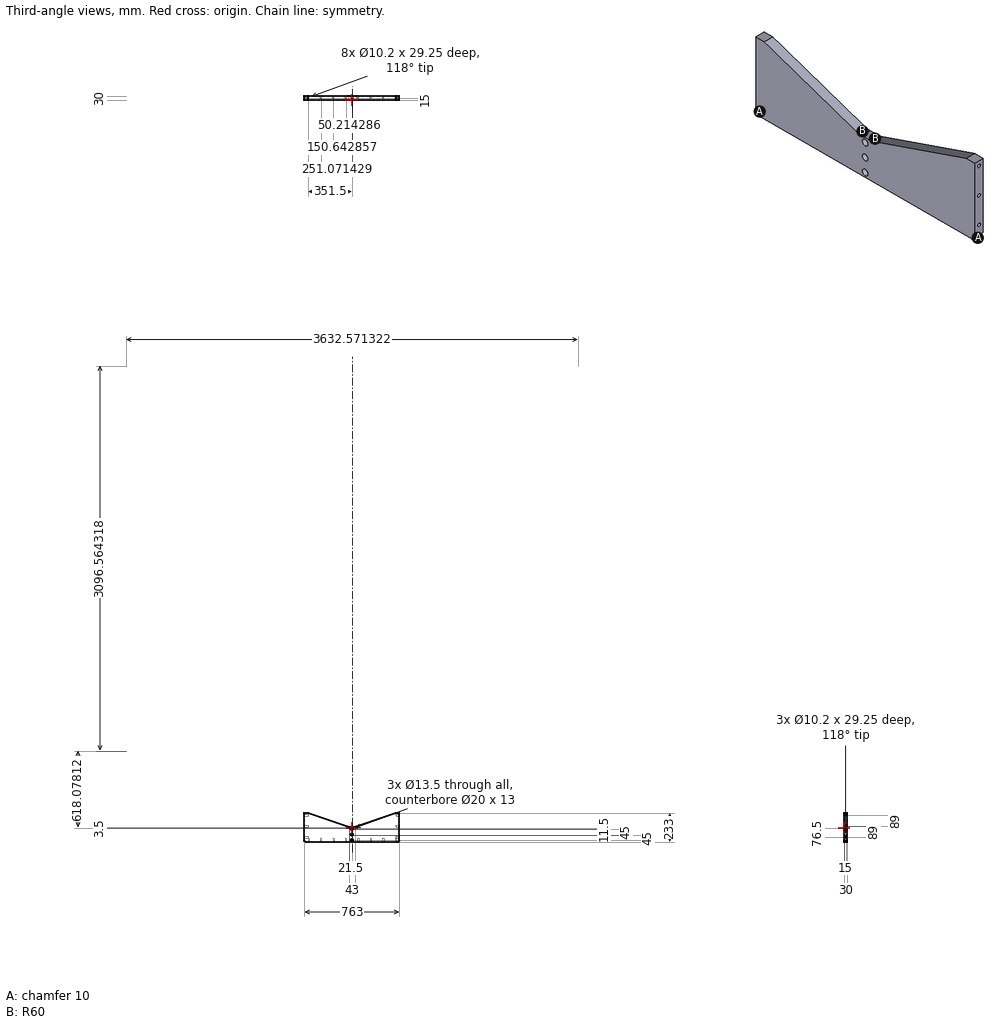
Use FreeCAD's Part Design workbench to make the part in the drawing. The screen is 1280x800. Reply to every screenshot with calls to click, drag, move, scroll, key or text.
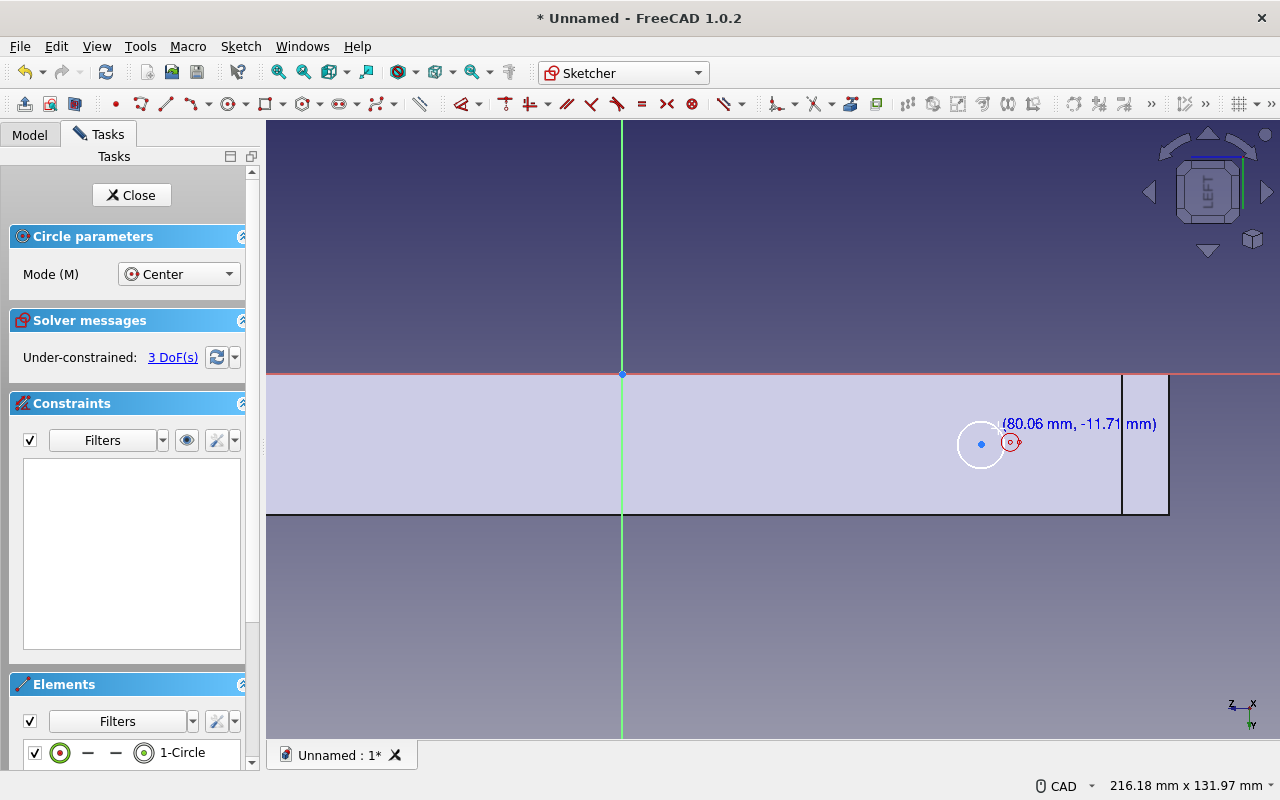
click(564, 444)
click(581, 428)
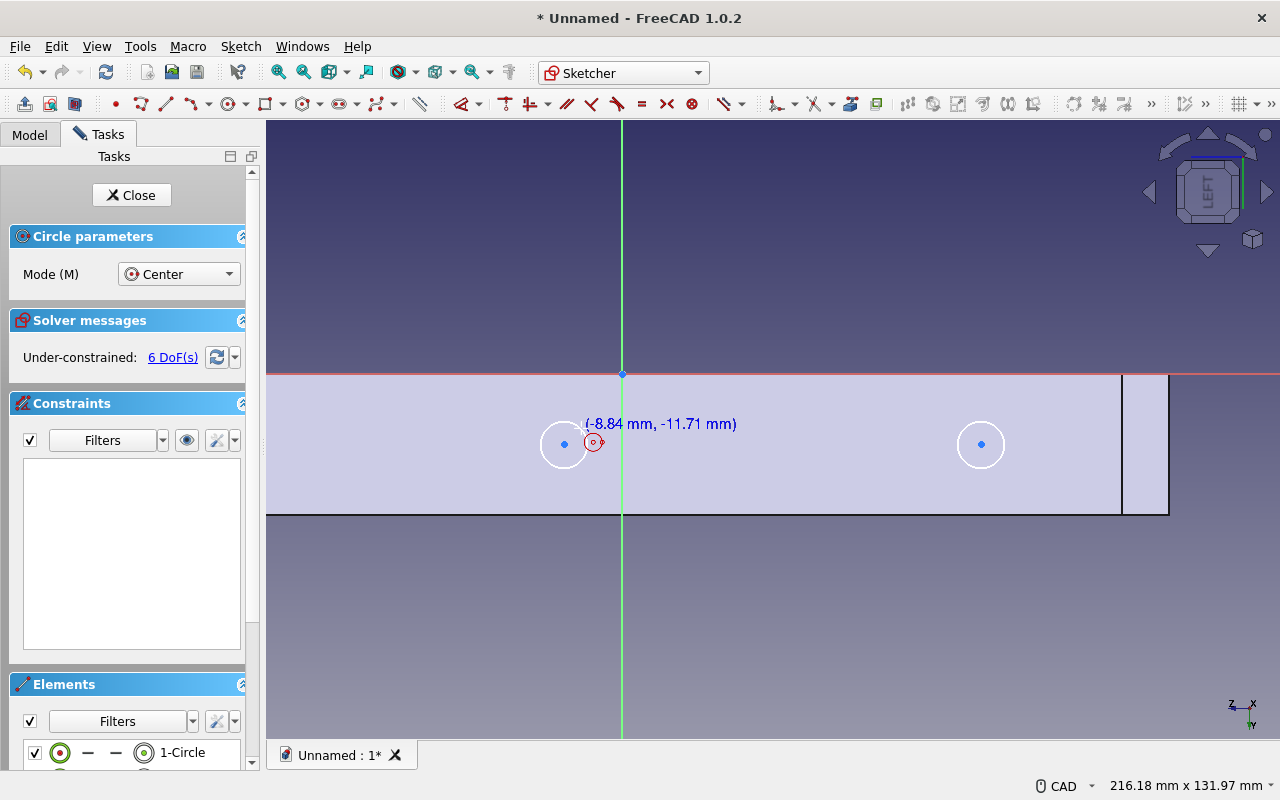
scroll(991, 446, down, 2)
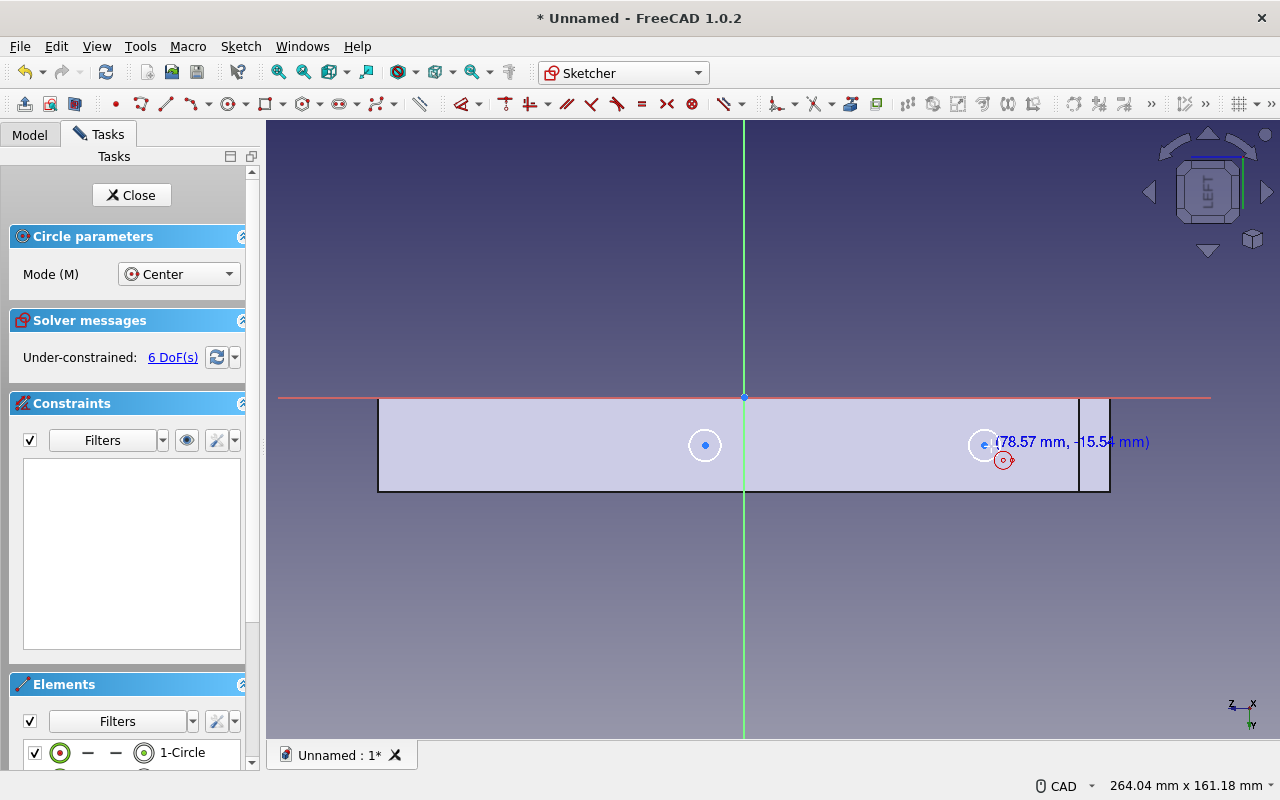
scroll(425, 445, up, 2)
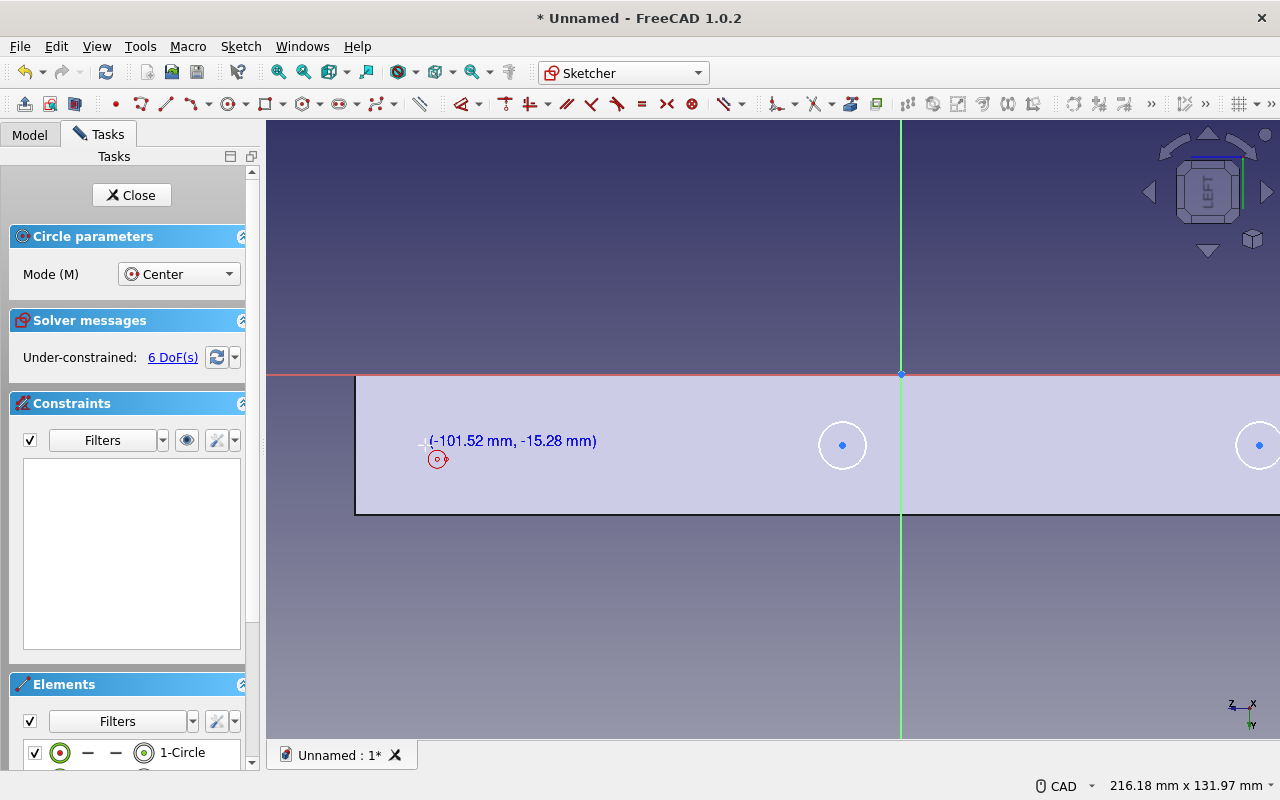
click(425, 445)
click(442, 428)
key(Escape)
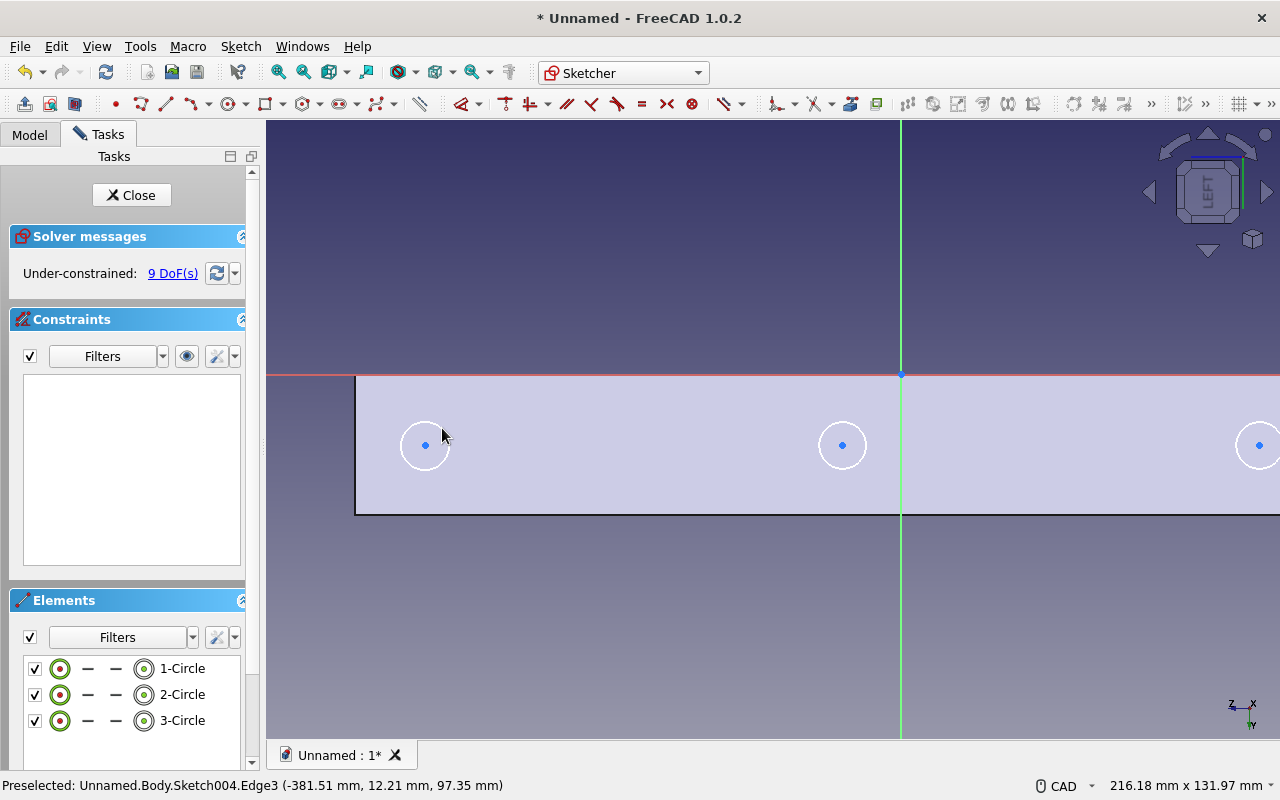
scroll(424, 445, down, 2)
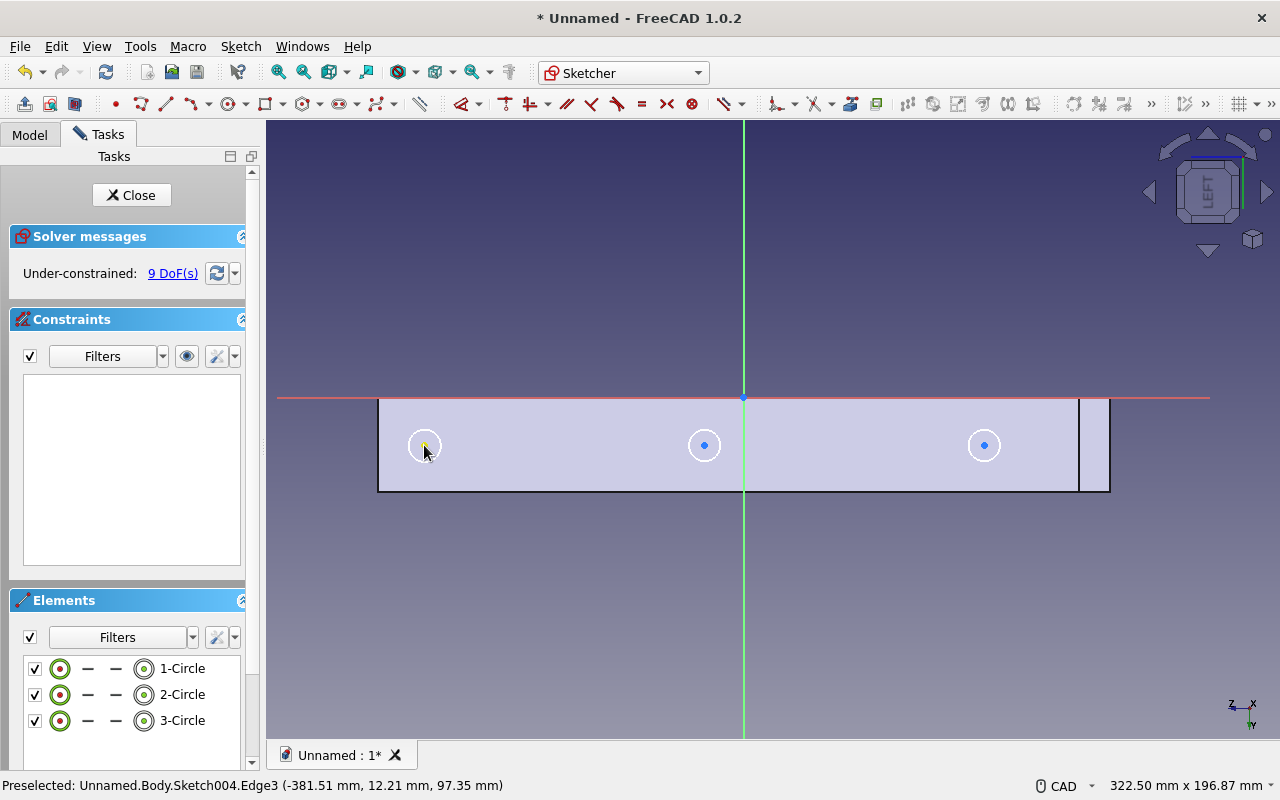
click(995, 434)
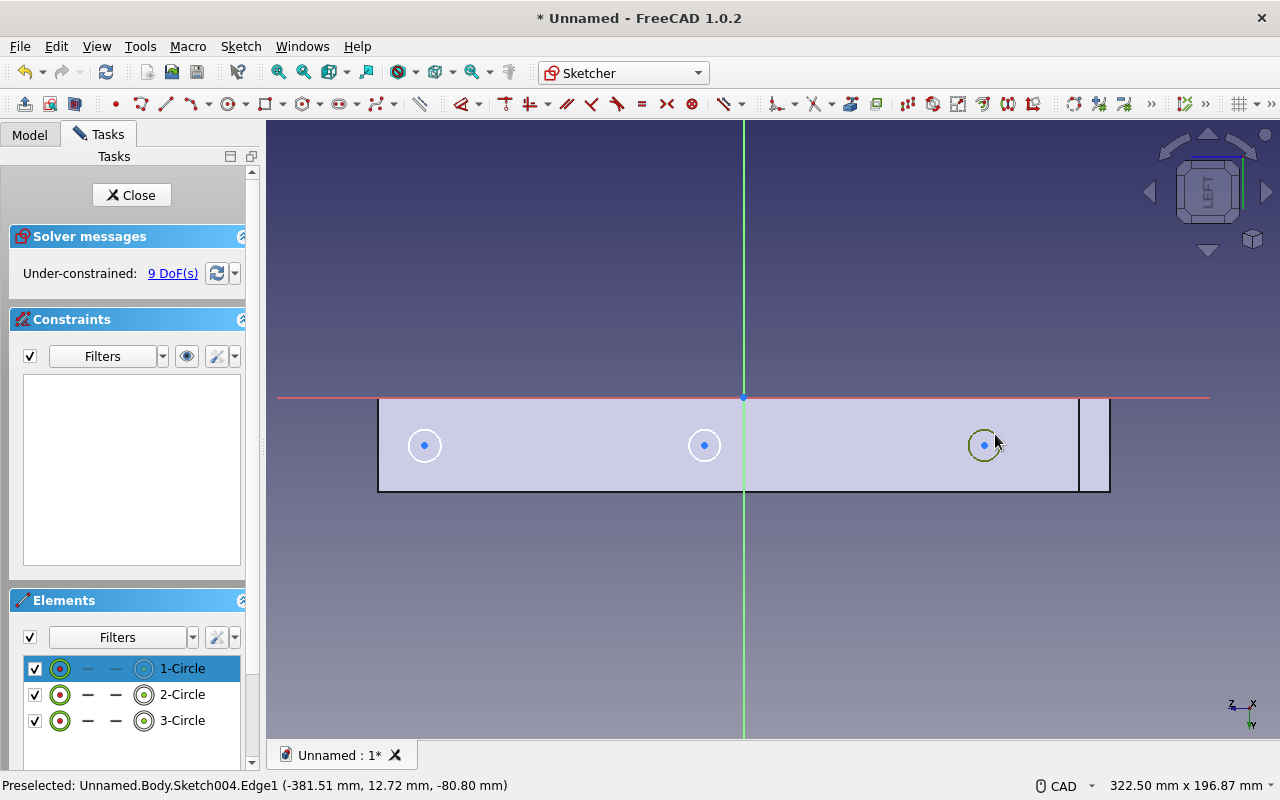
click(716, 434)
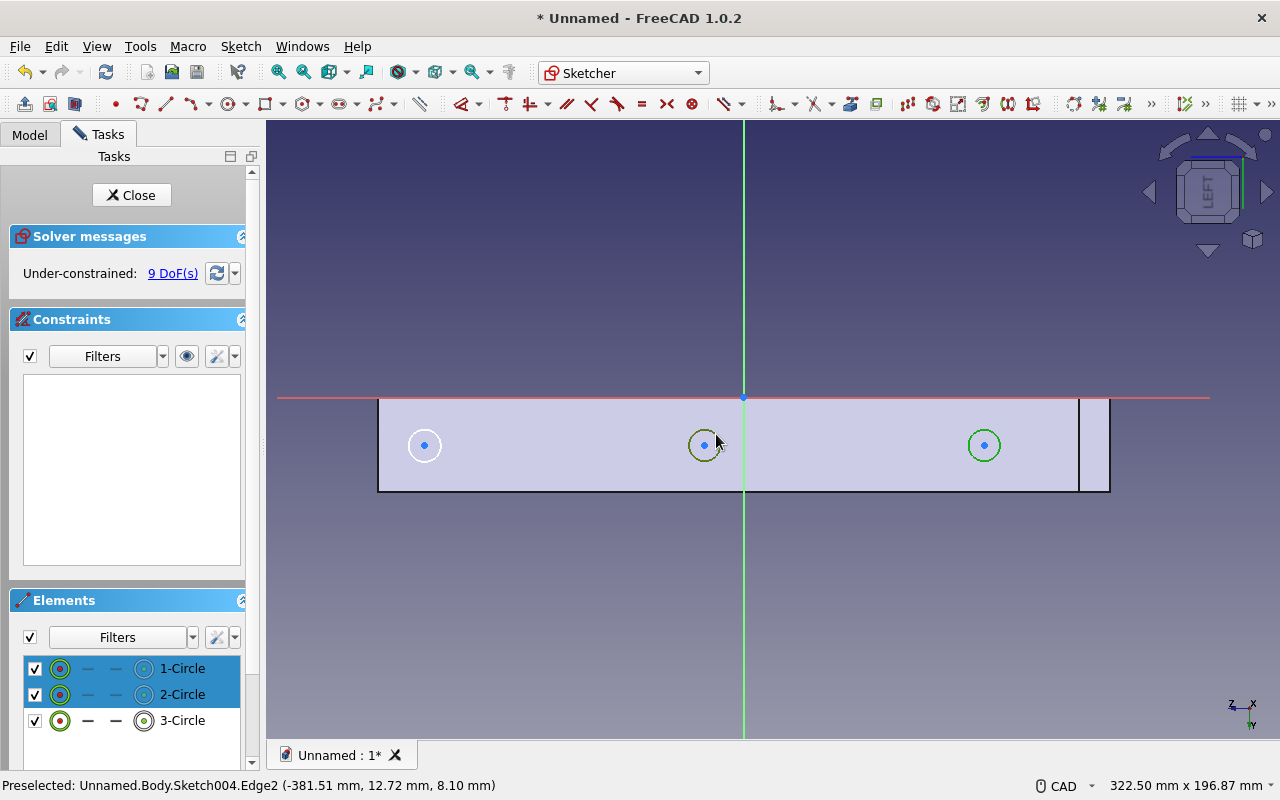
click(436, 434)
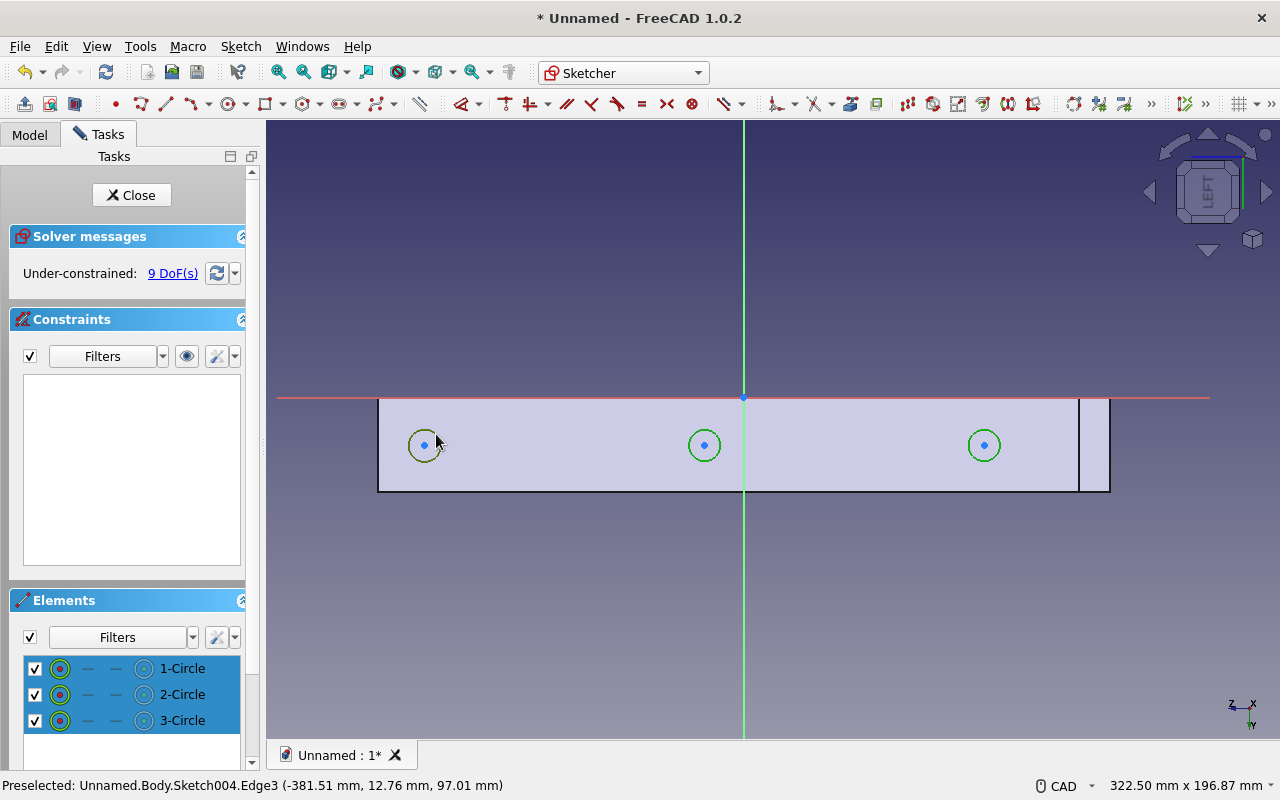
key(e)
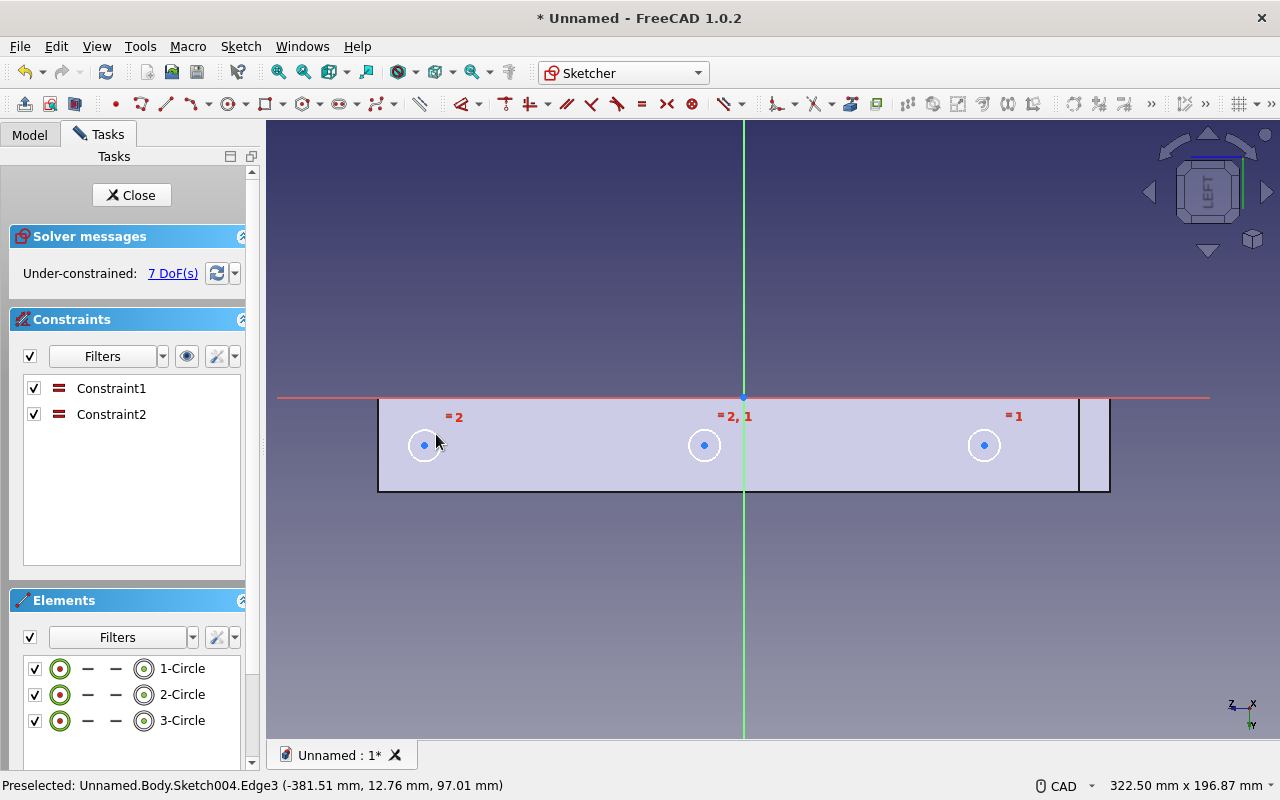
key(d)